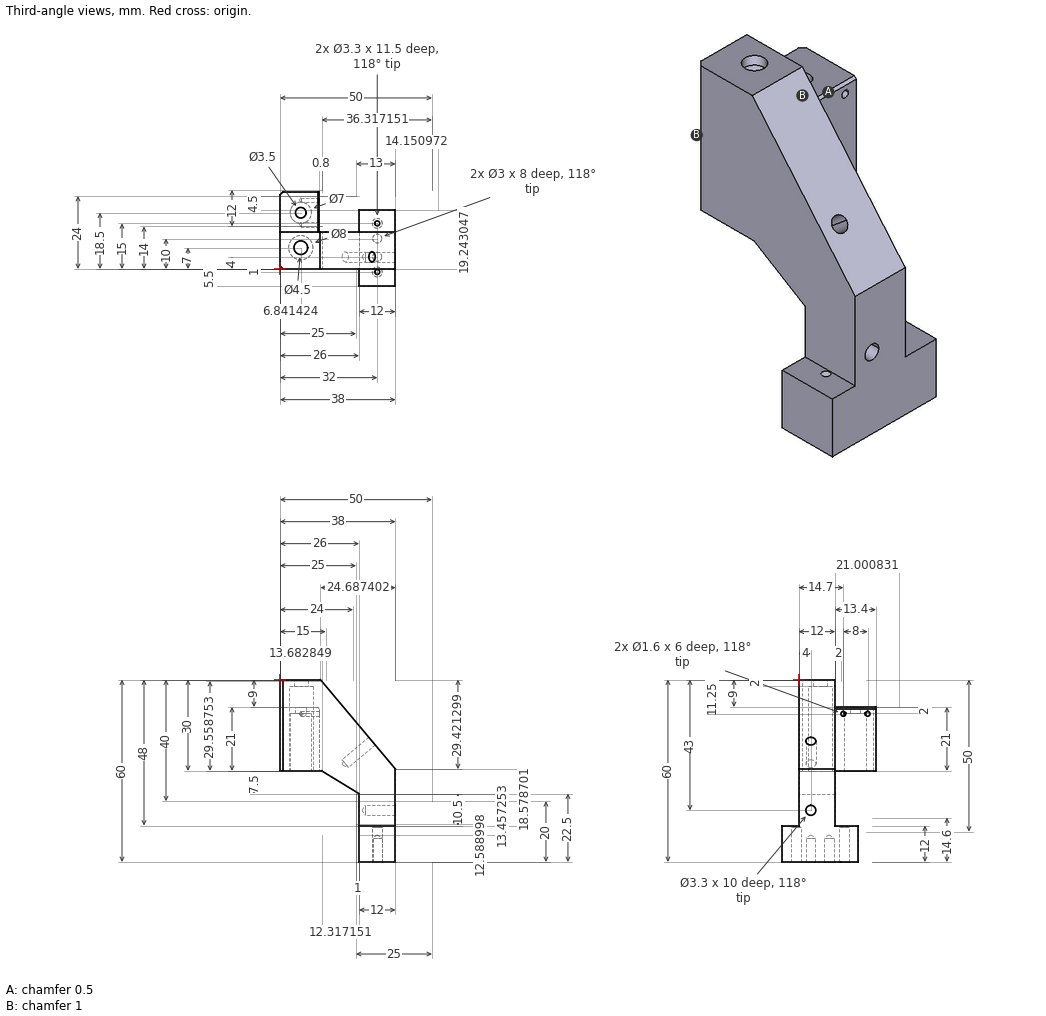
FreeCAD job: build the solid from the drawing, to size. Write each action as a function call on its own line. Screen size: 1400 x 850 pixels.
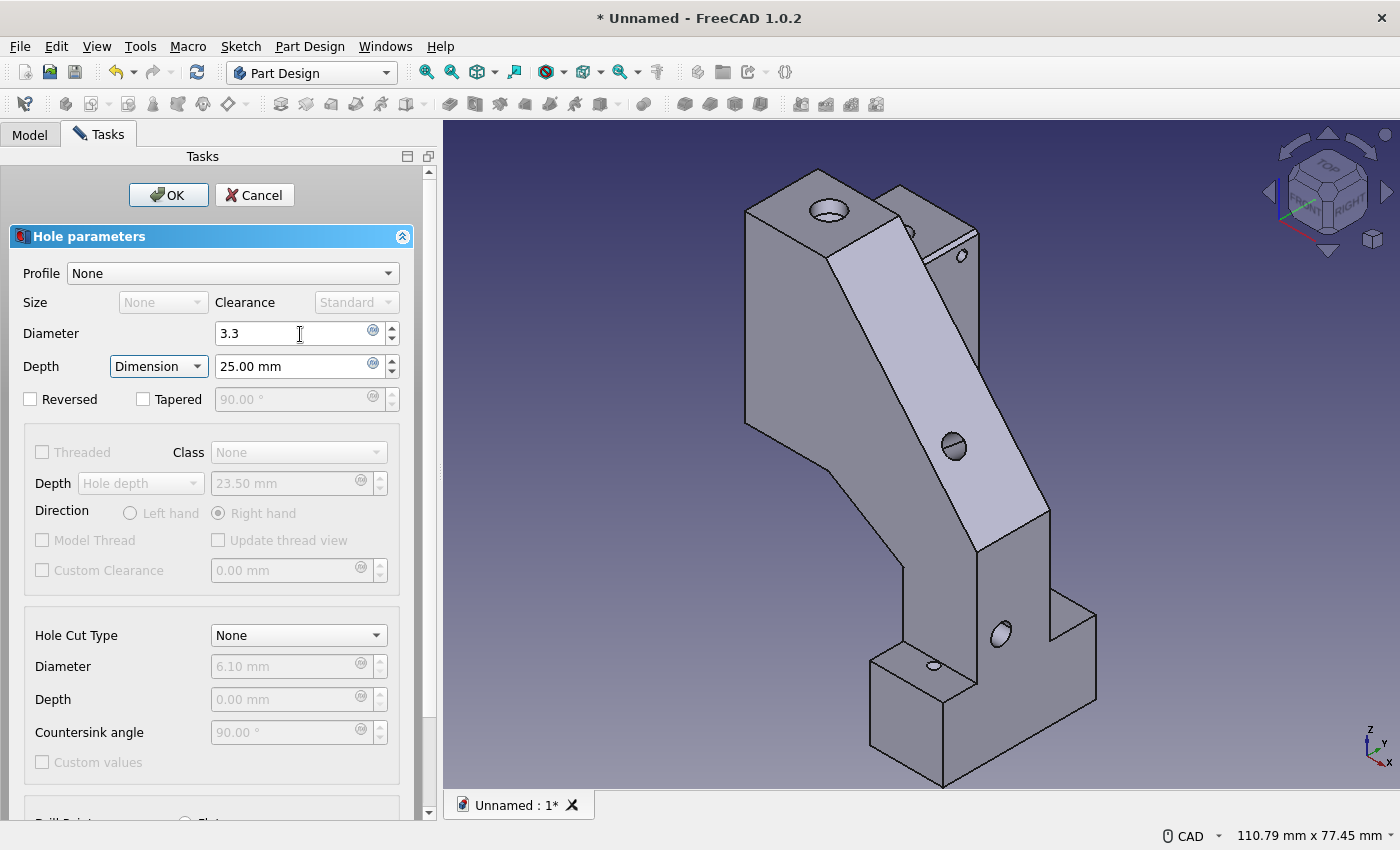
triple_click(300, 366)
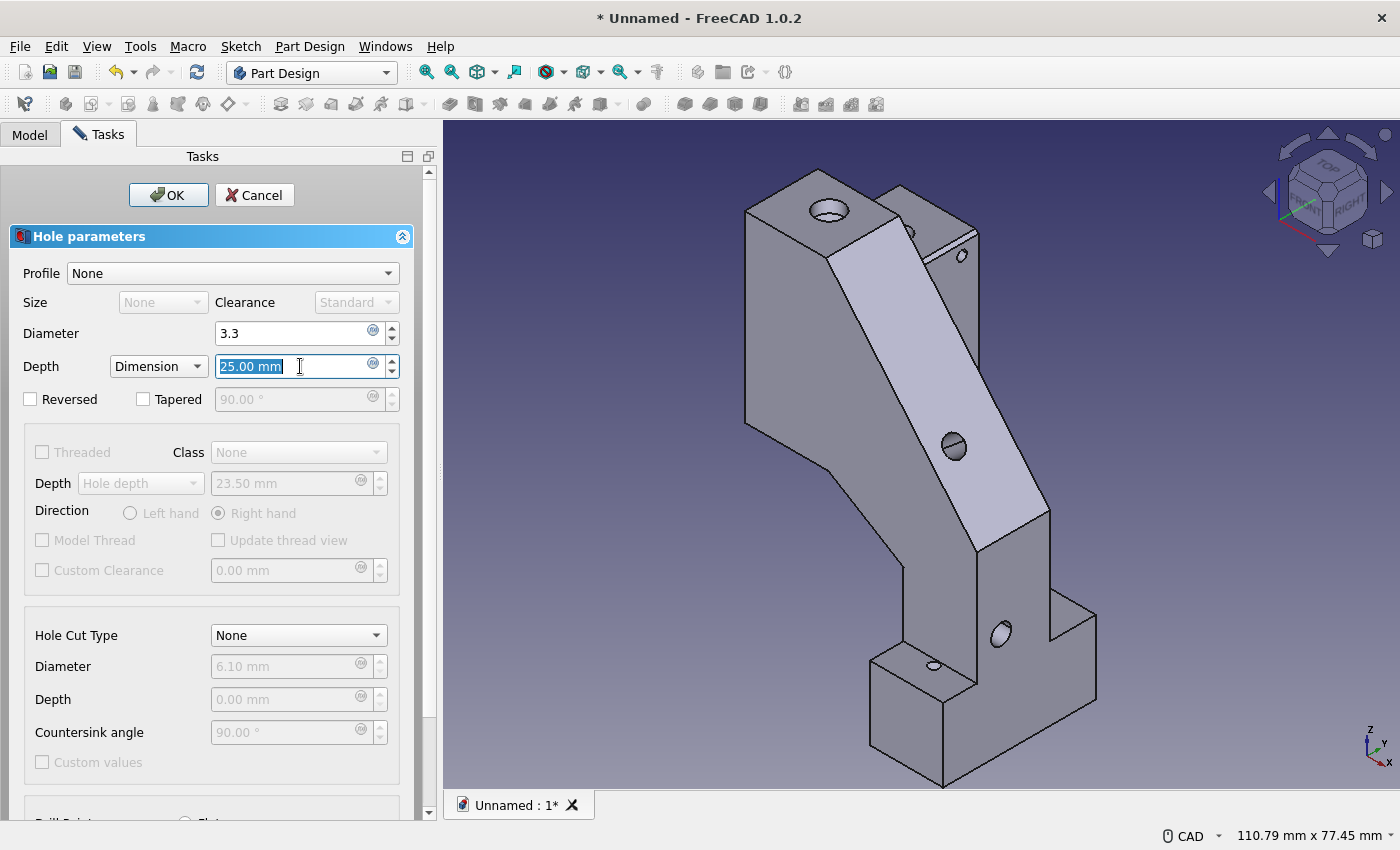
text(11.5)
key(Tab)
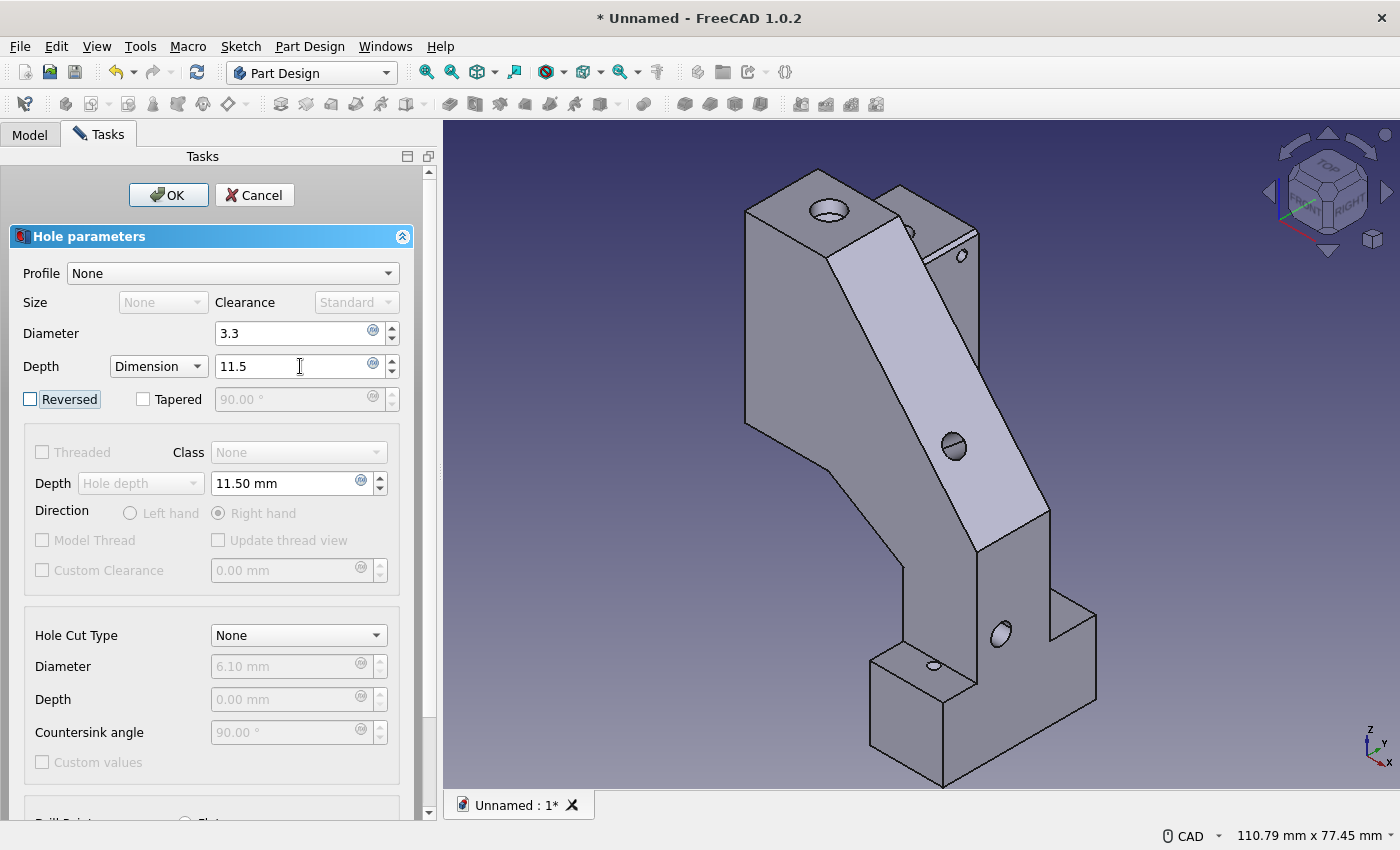
click(169, 195)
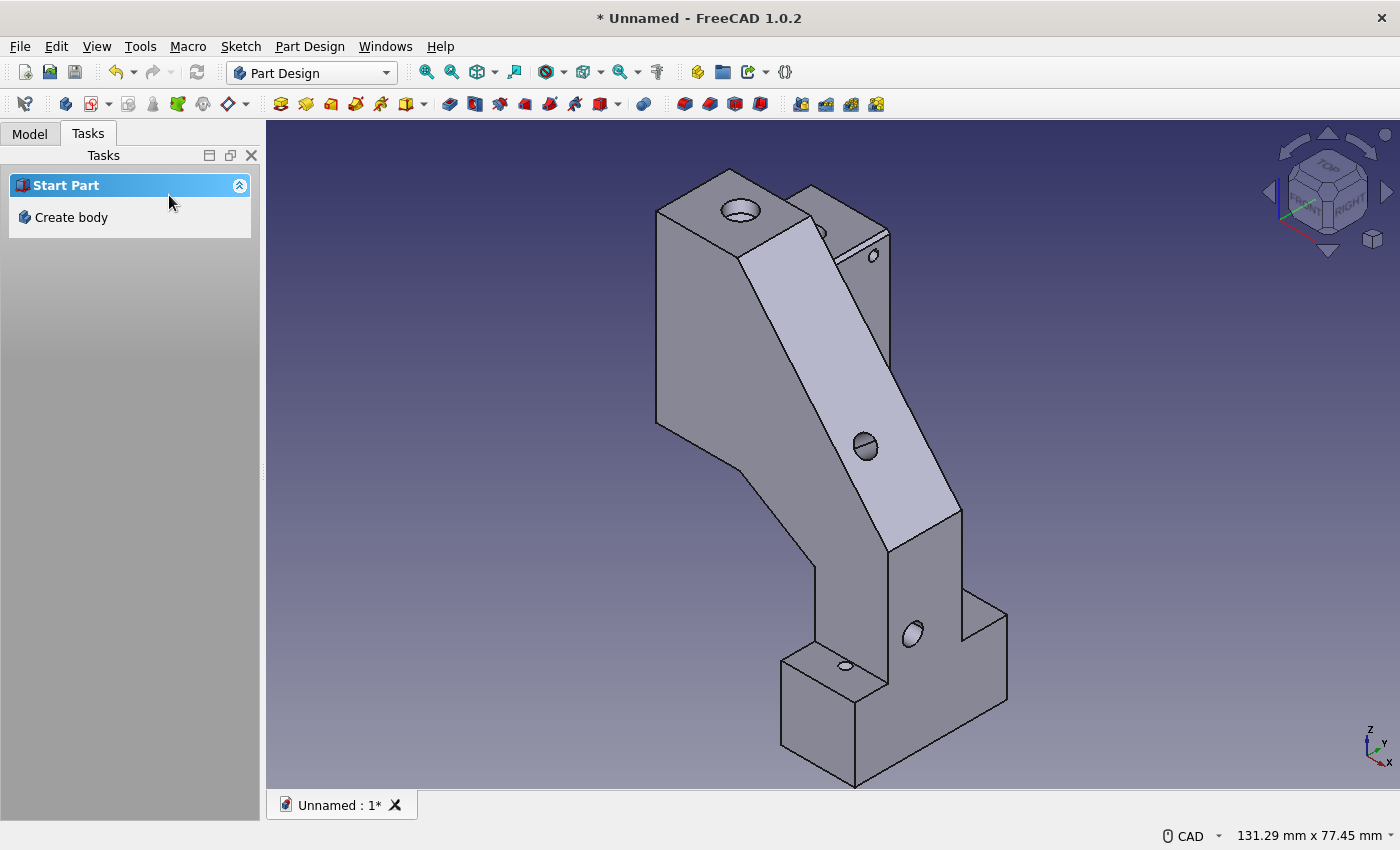
key(2)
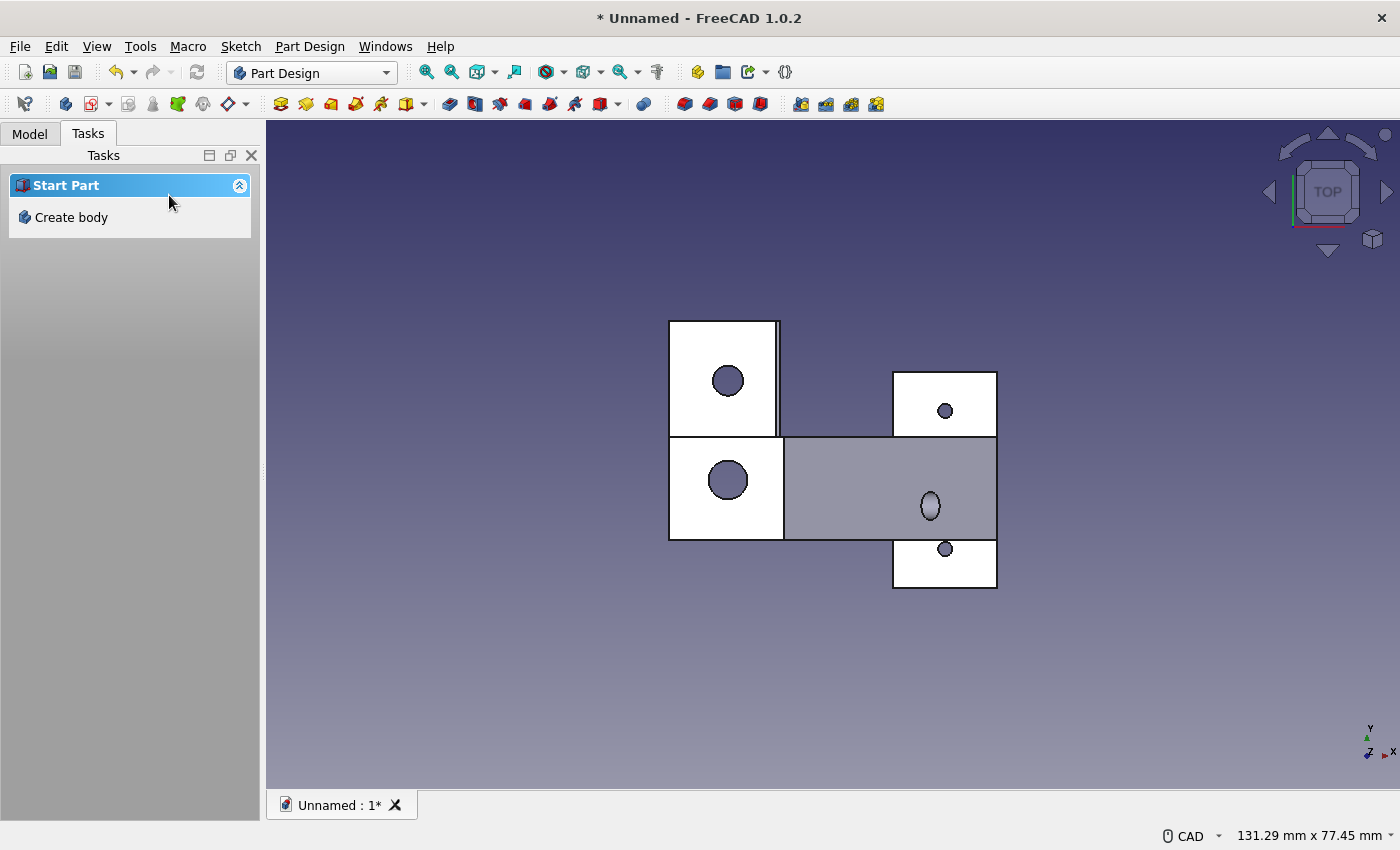
click(427, 72)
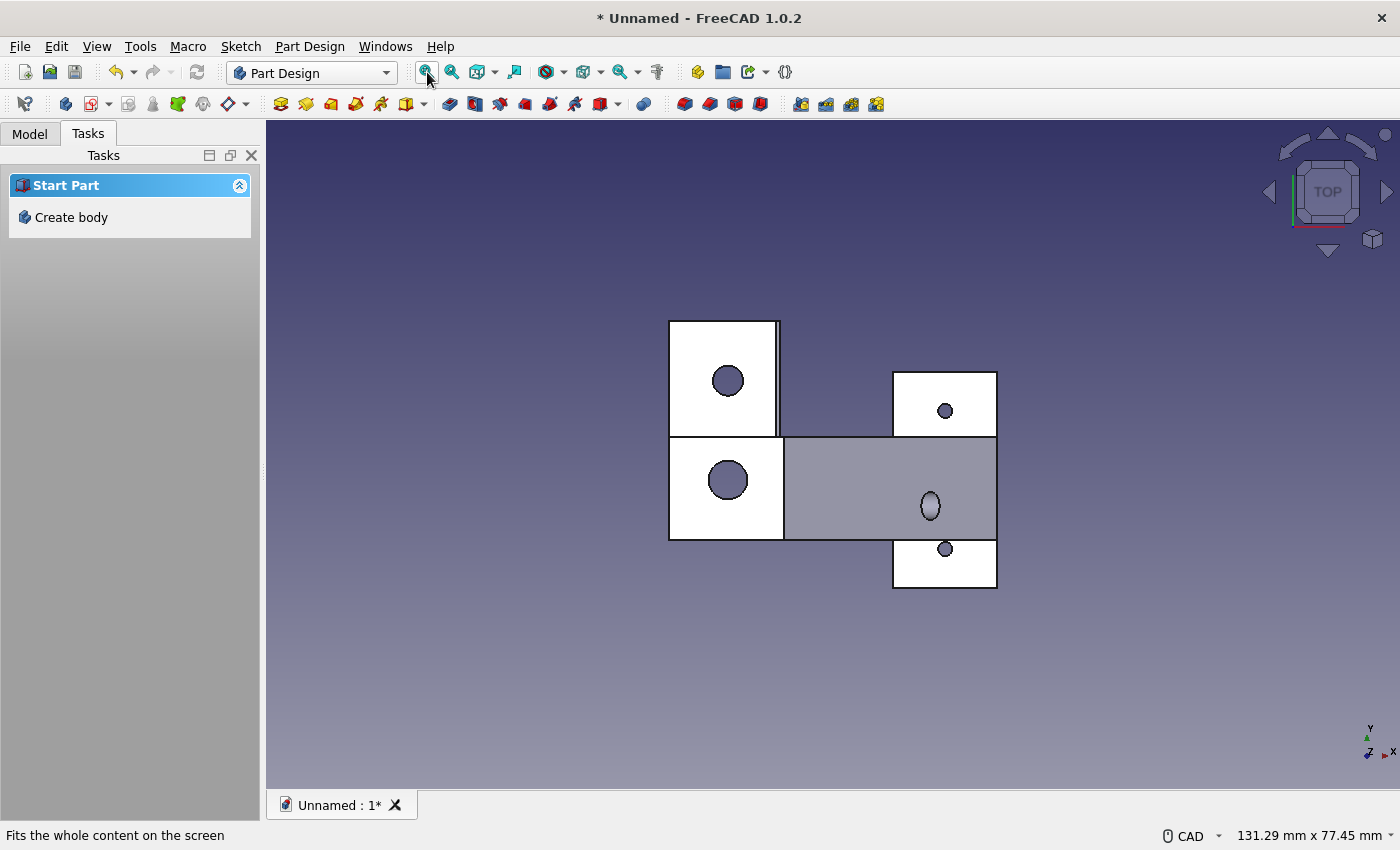
key(0)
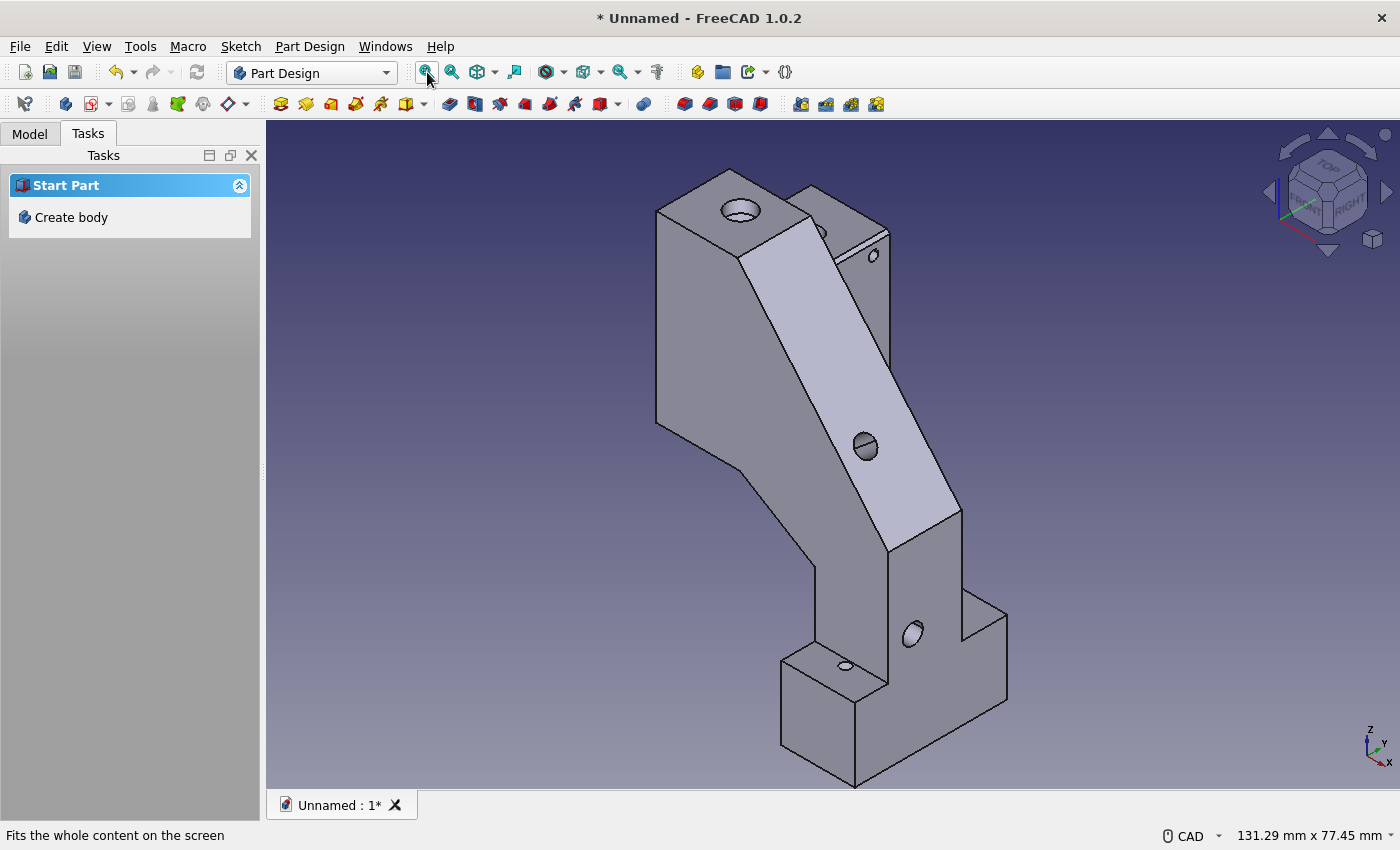
key(1)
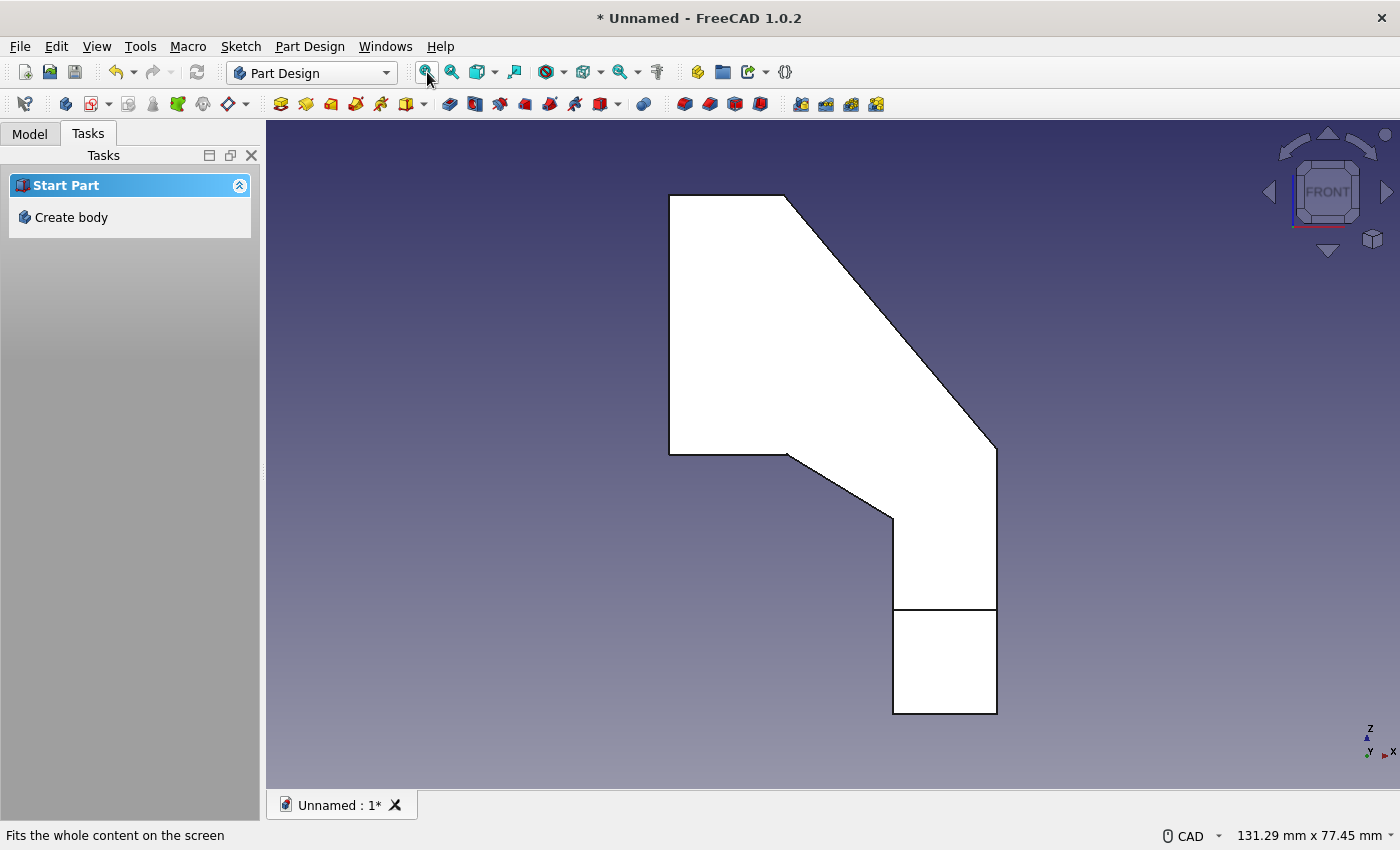
click(669, 272)